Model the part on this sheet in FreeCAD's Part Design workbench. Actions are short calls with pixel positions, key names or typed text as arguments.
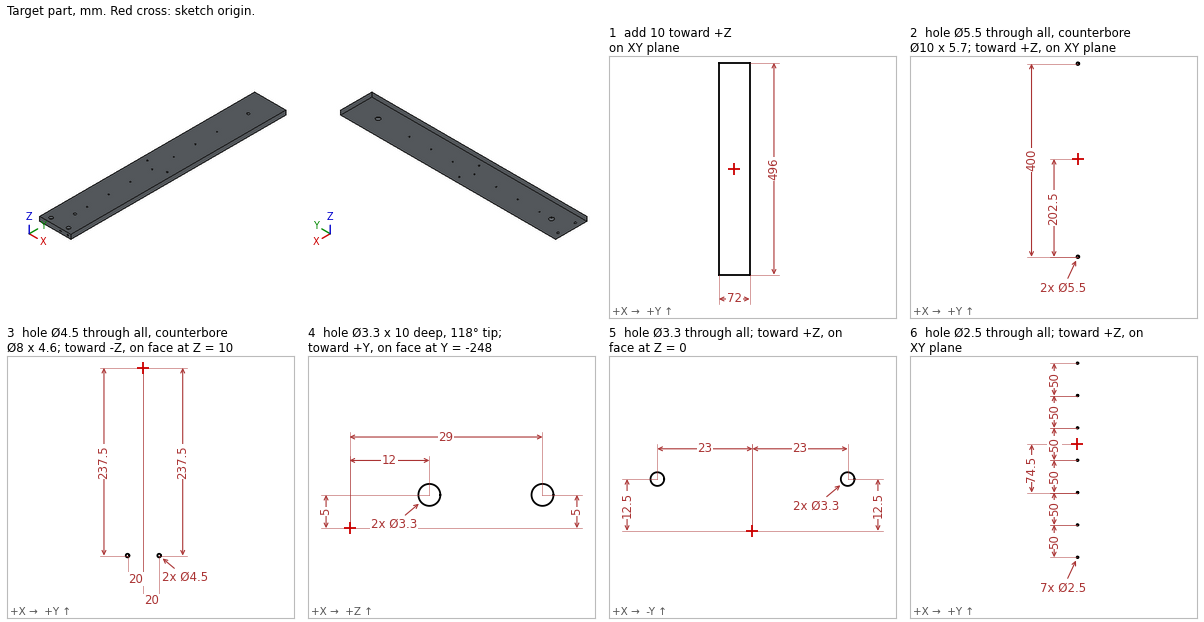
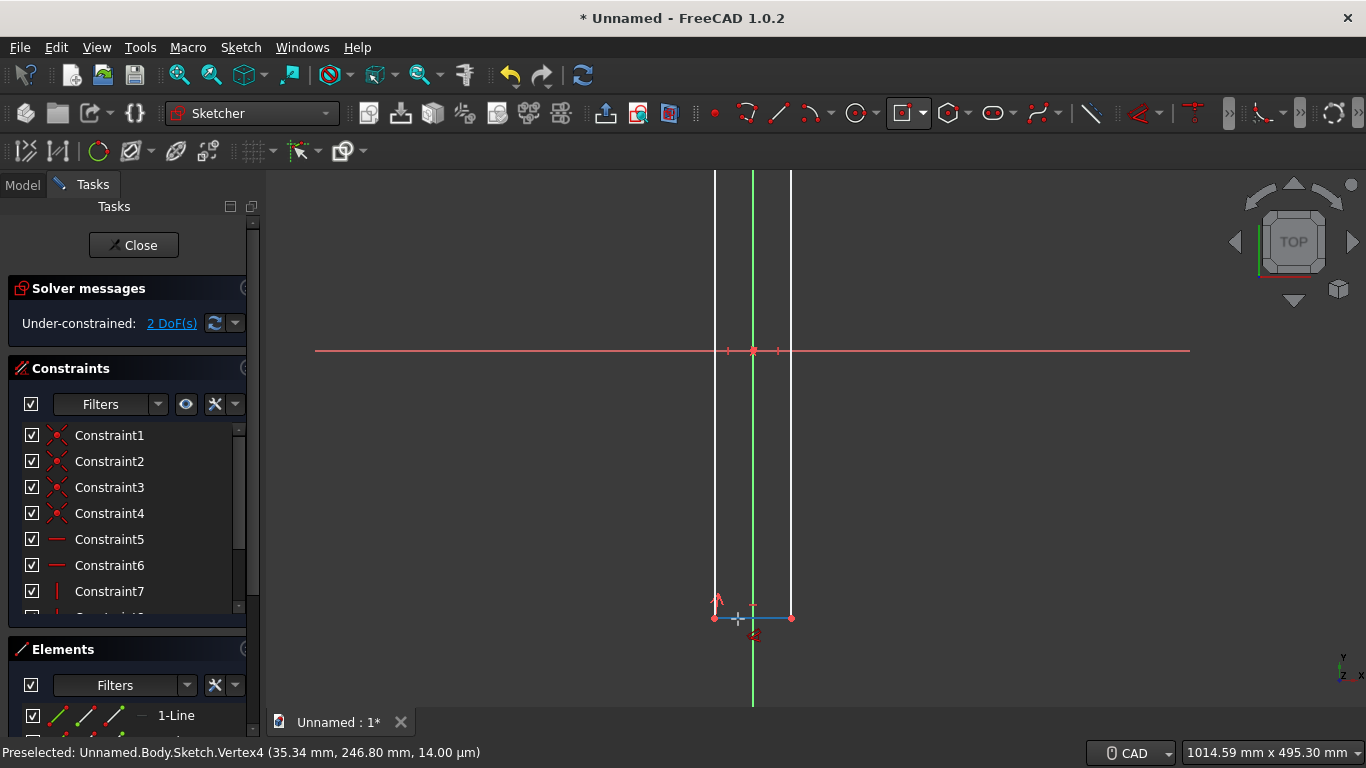
click(738, 618)
click(736, 652)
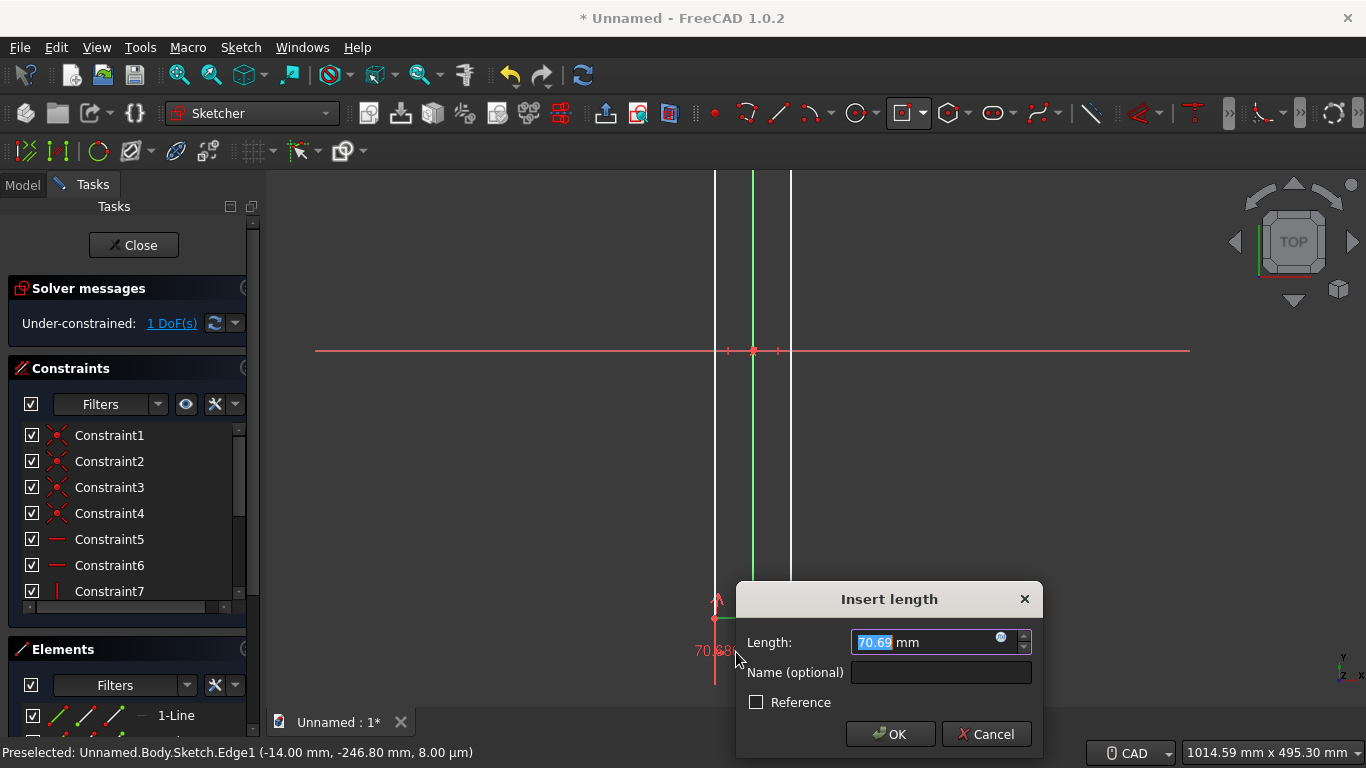
text(72)
key(Return)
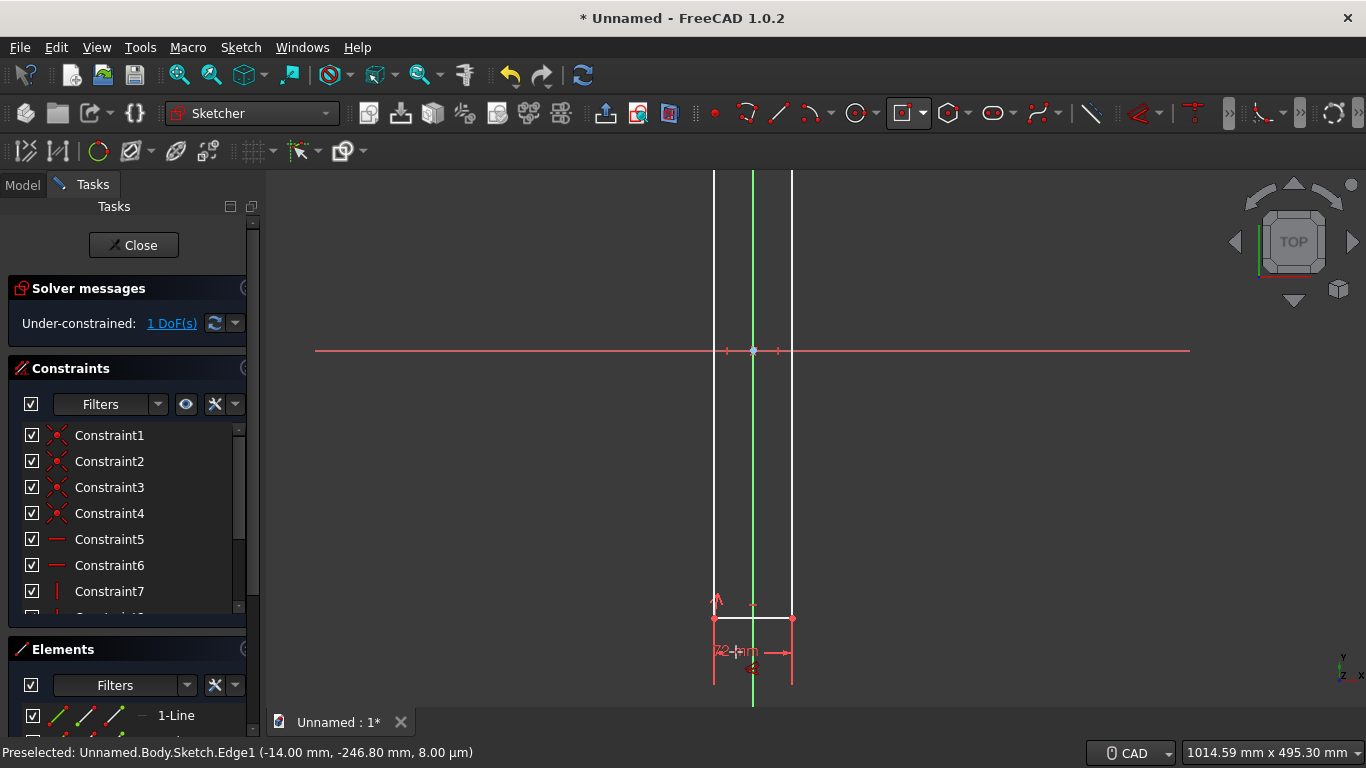
click(792, 458)
click(826, 408)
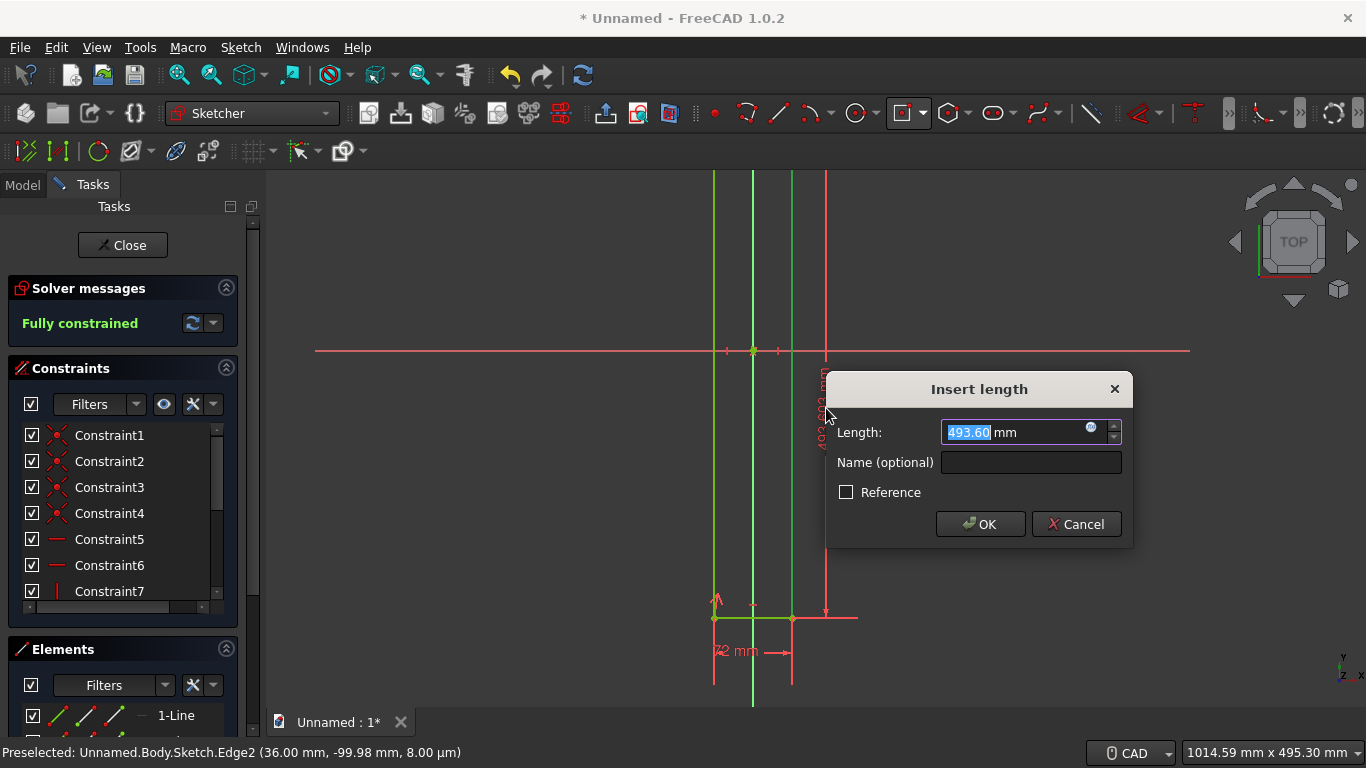
text(496)
key(Return)
key(Escape)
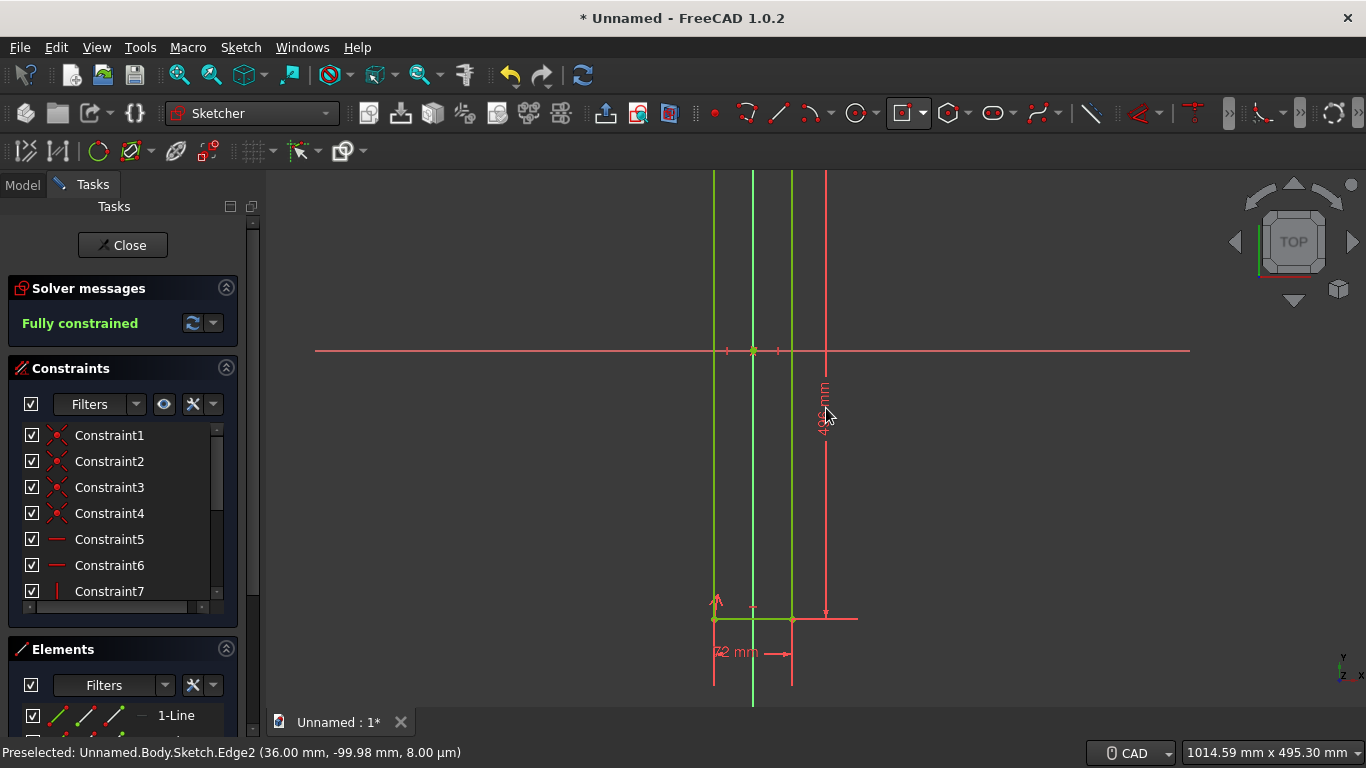
click(123, 245)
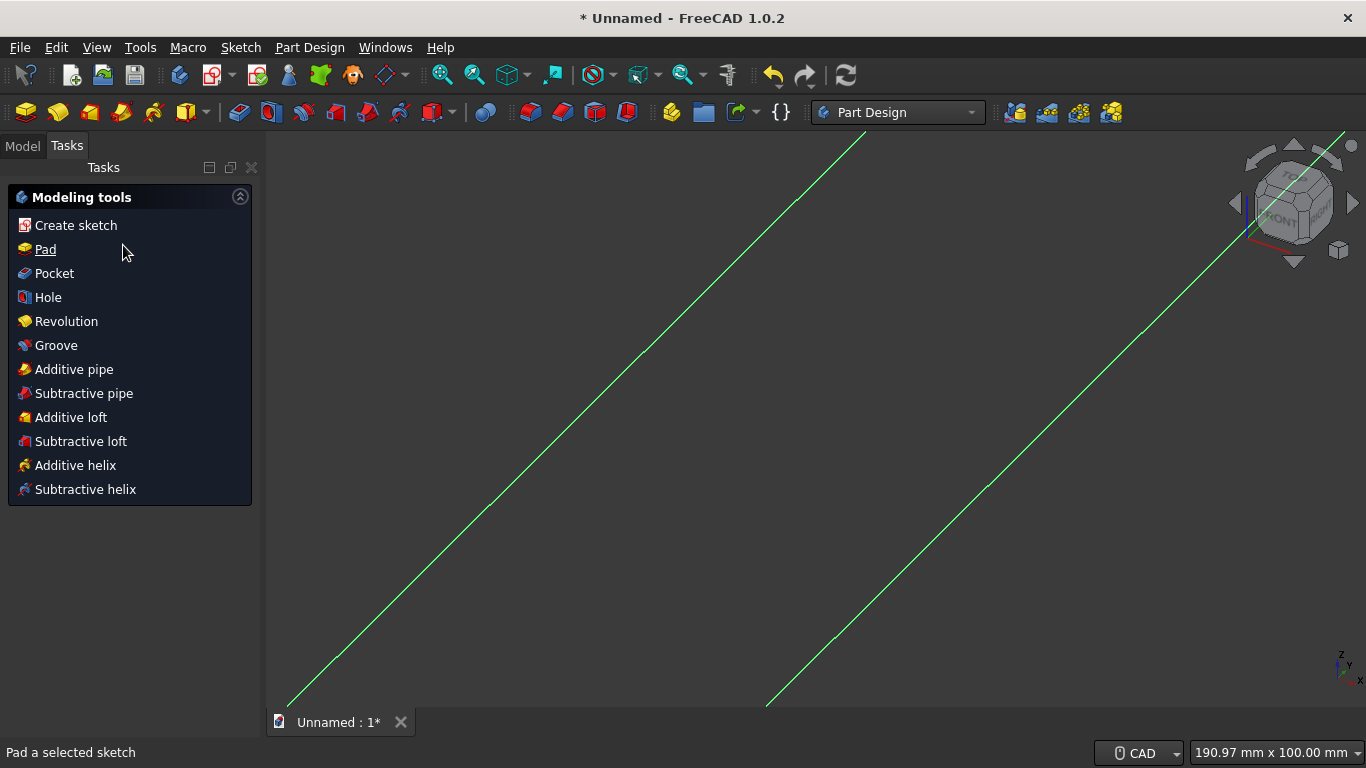
click(26, 112)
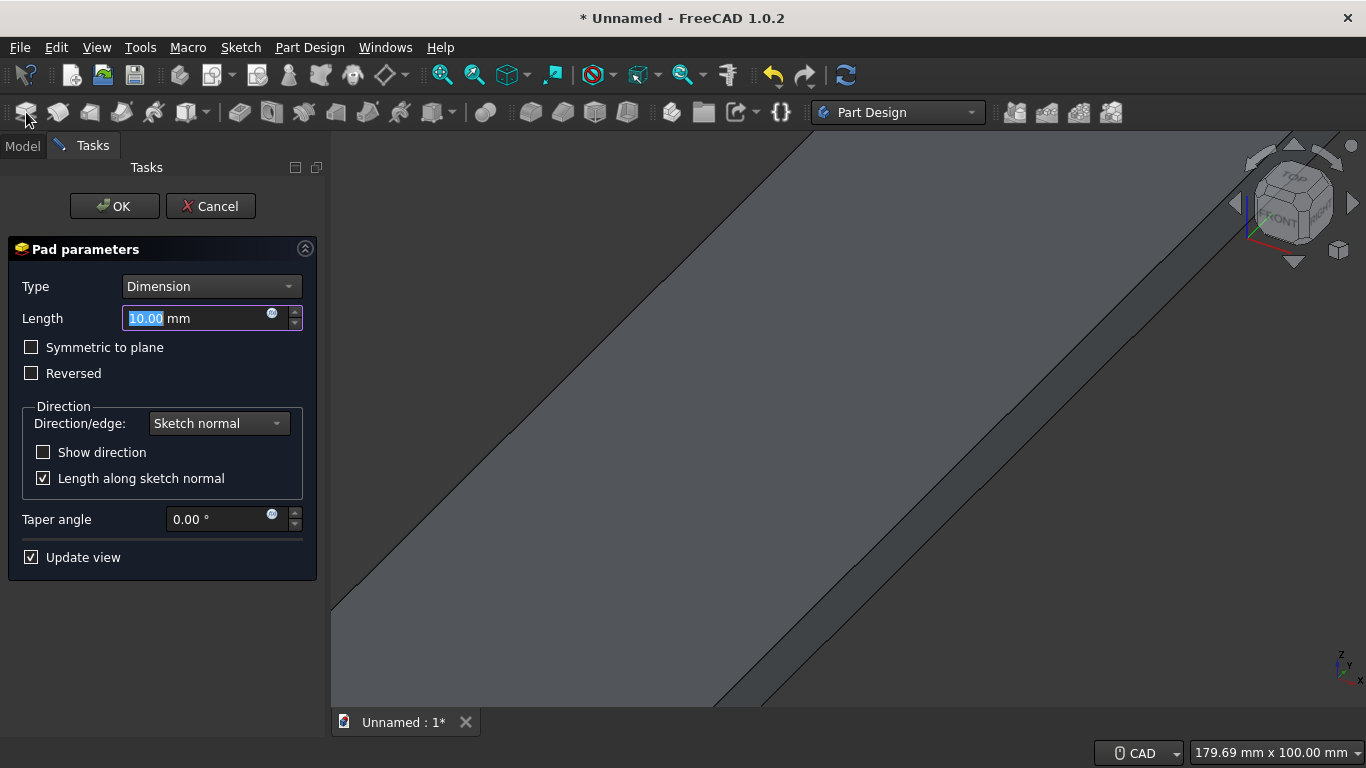
text(10)
key(Tab)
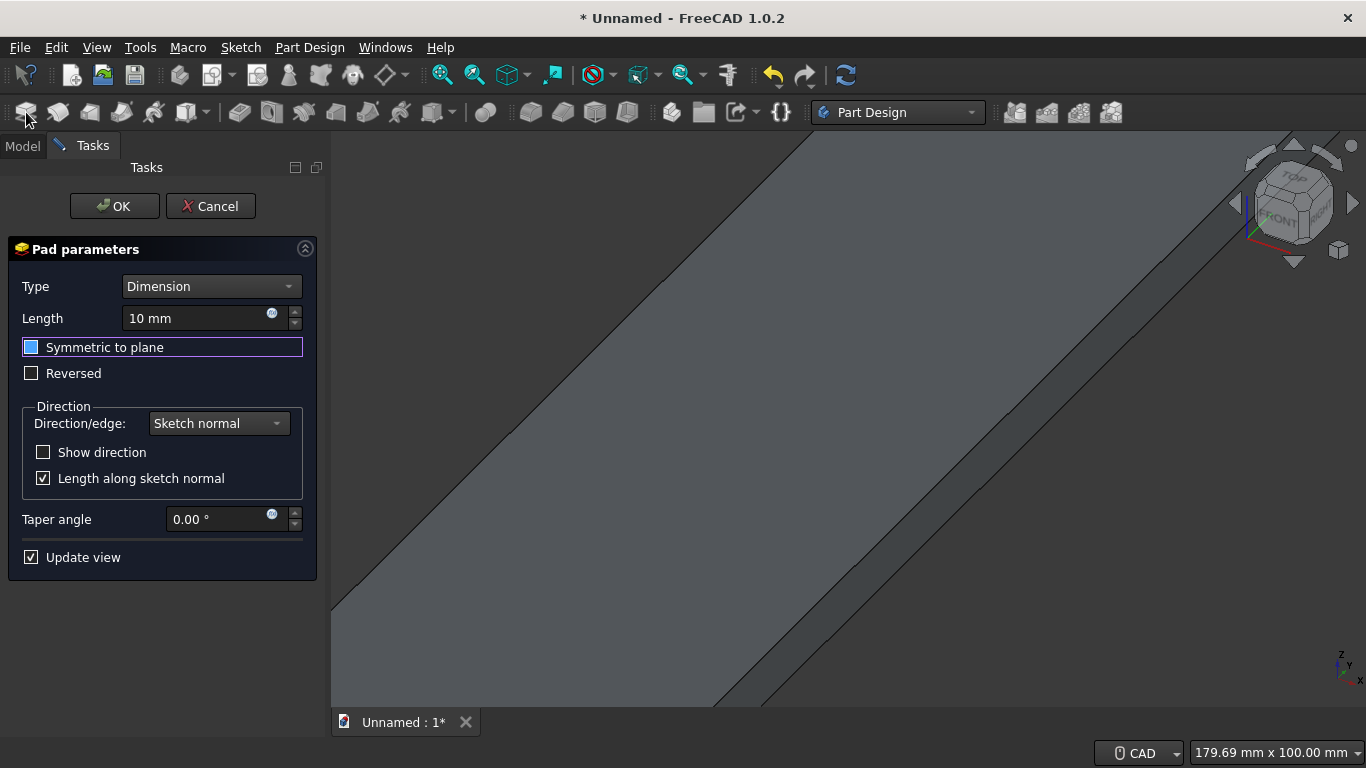
click(115, 206)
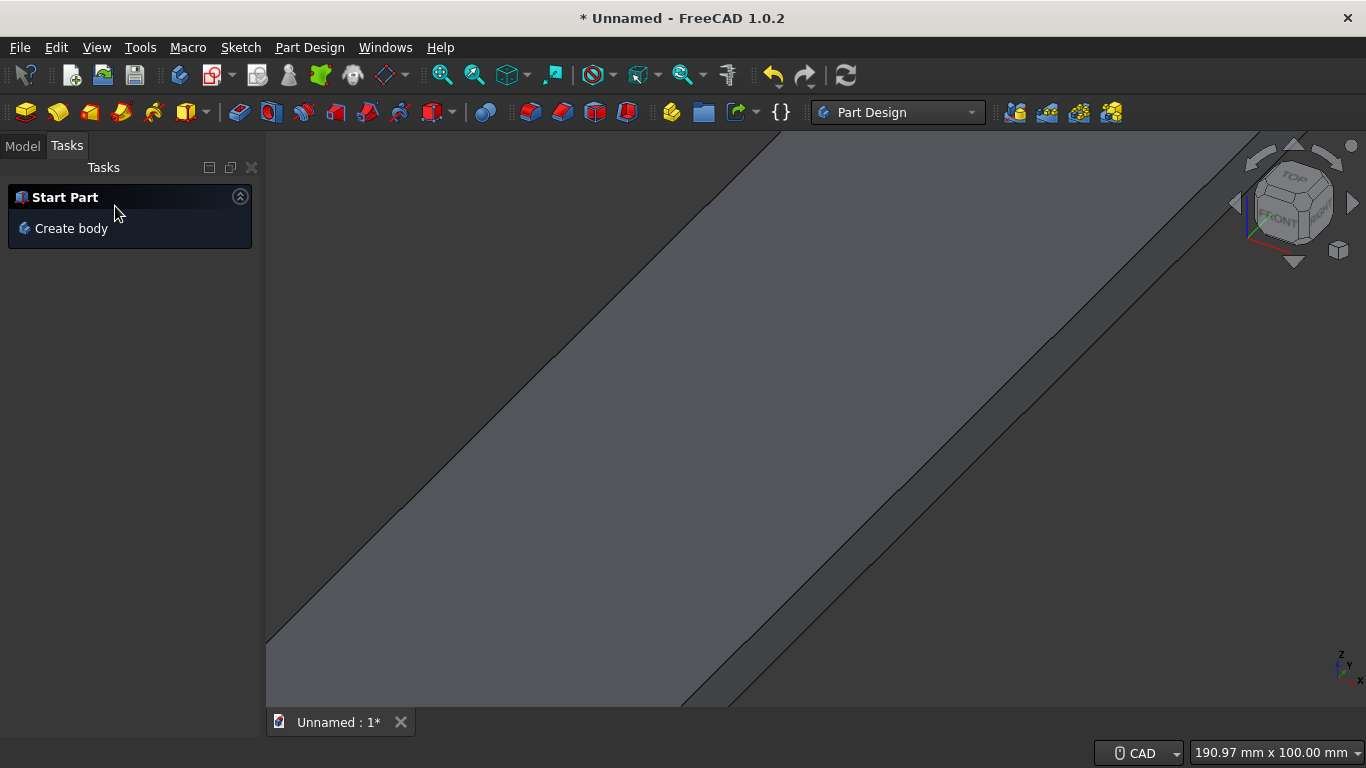
click(444, 76)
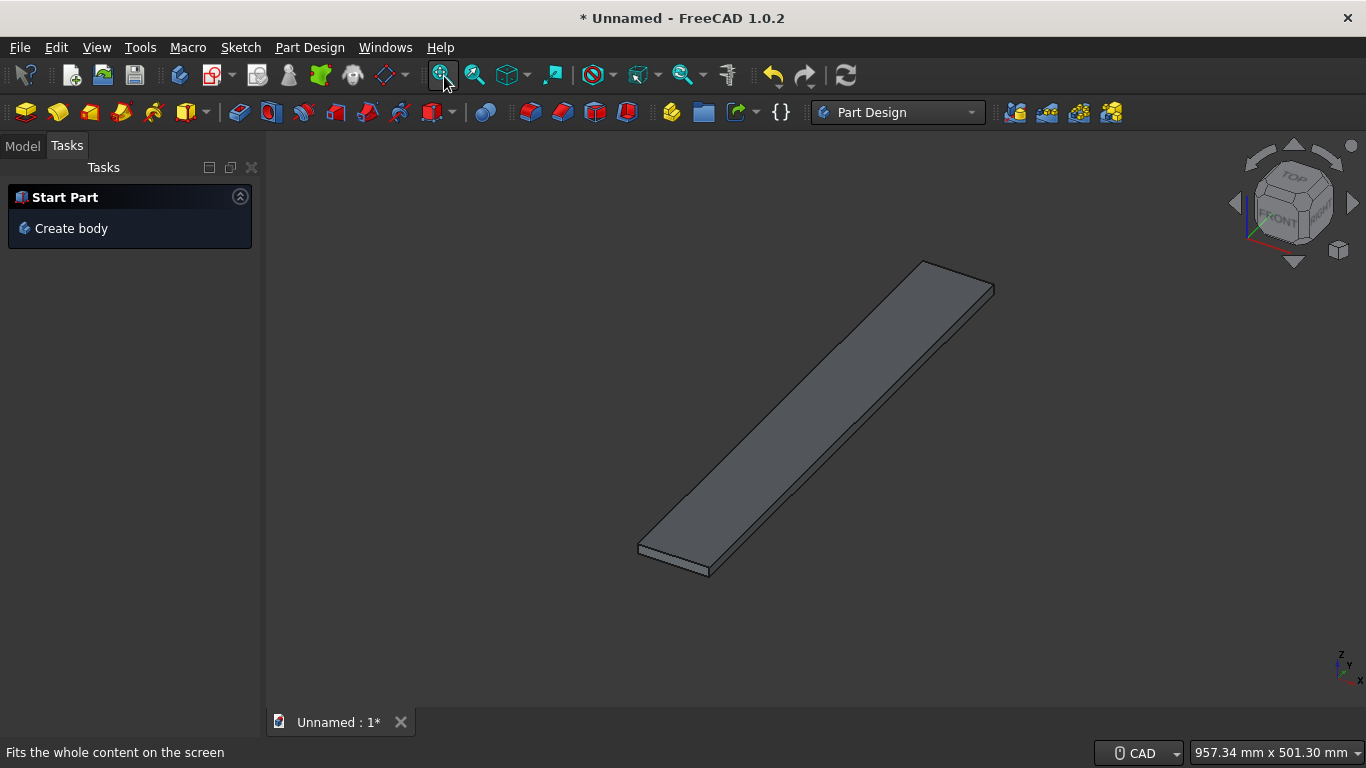
click(212, 76)